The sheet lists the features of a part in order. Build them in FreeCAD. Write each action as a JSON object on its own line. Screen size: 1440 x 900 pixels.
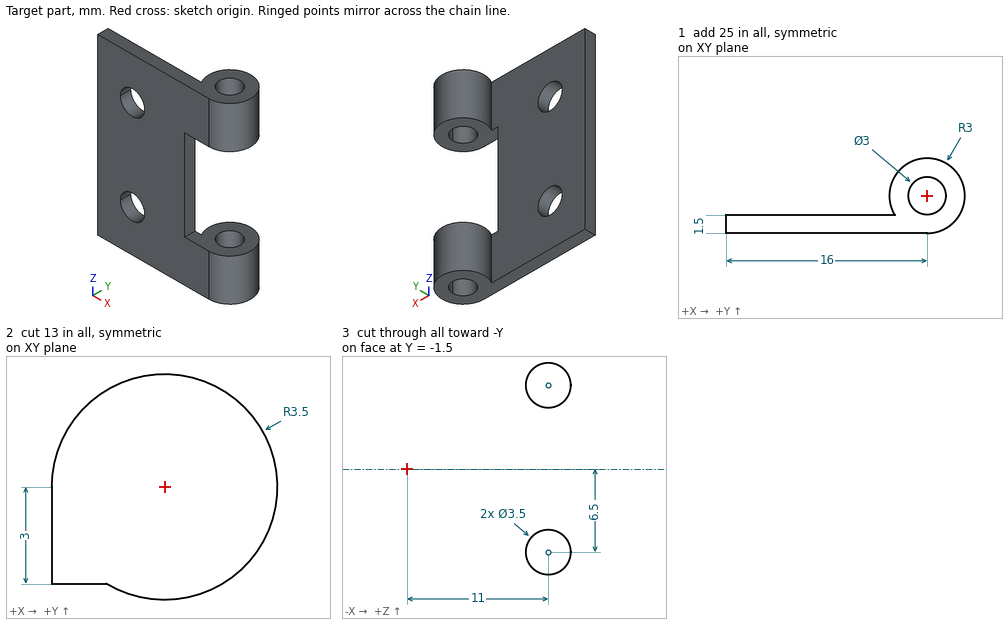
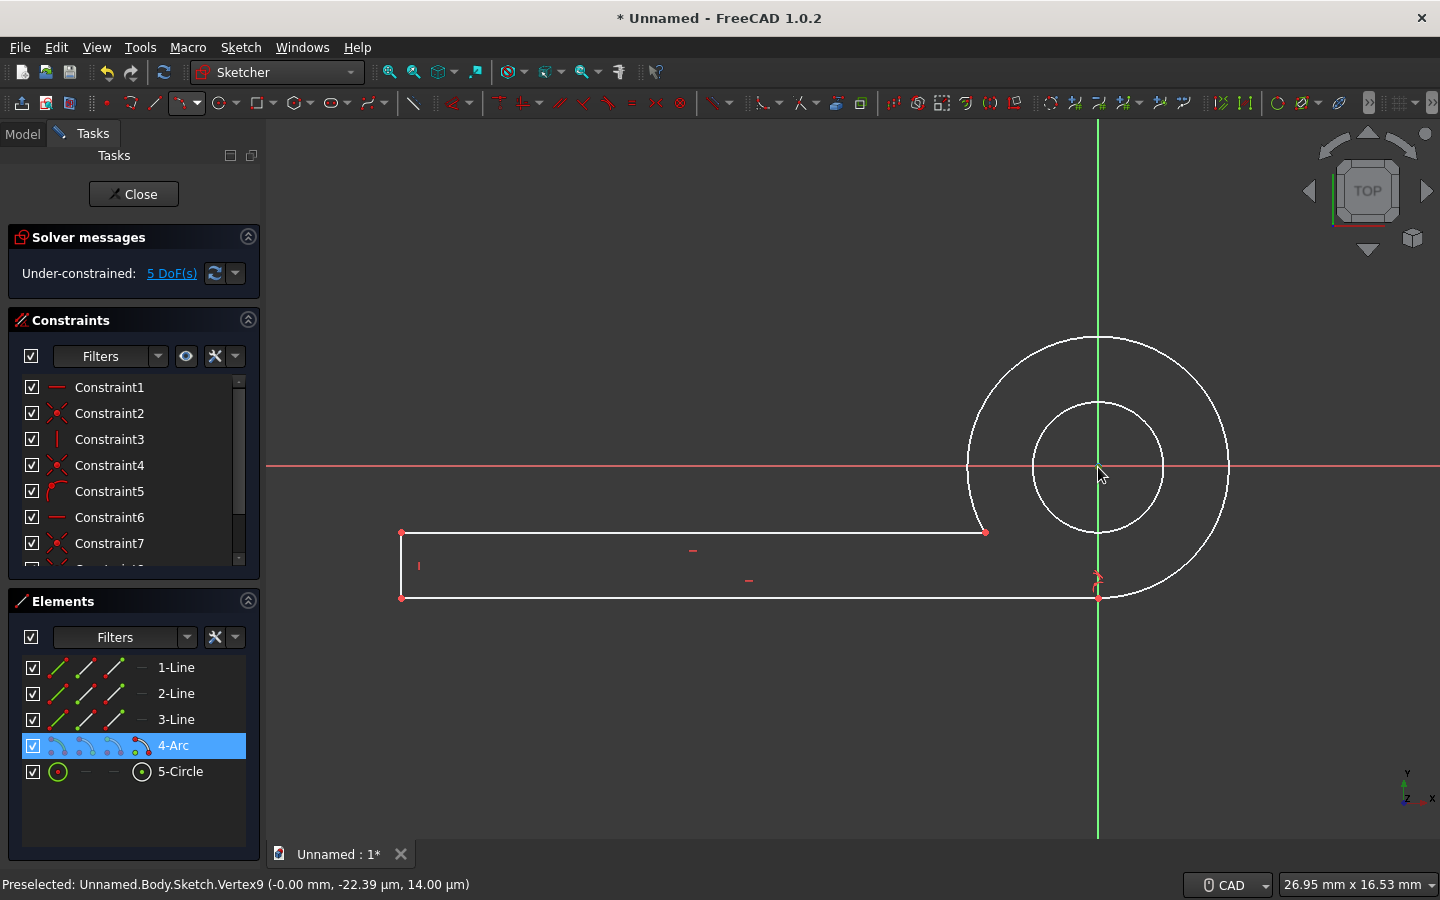
{"action": "left_click", "coordinate": [364, 466]}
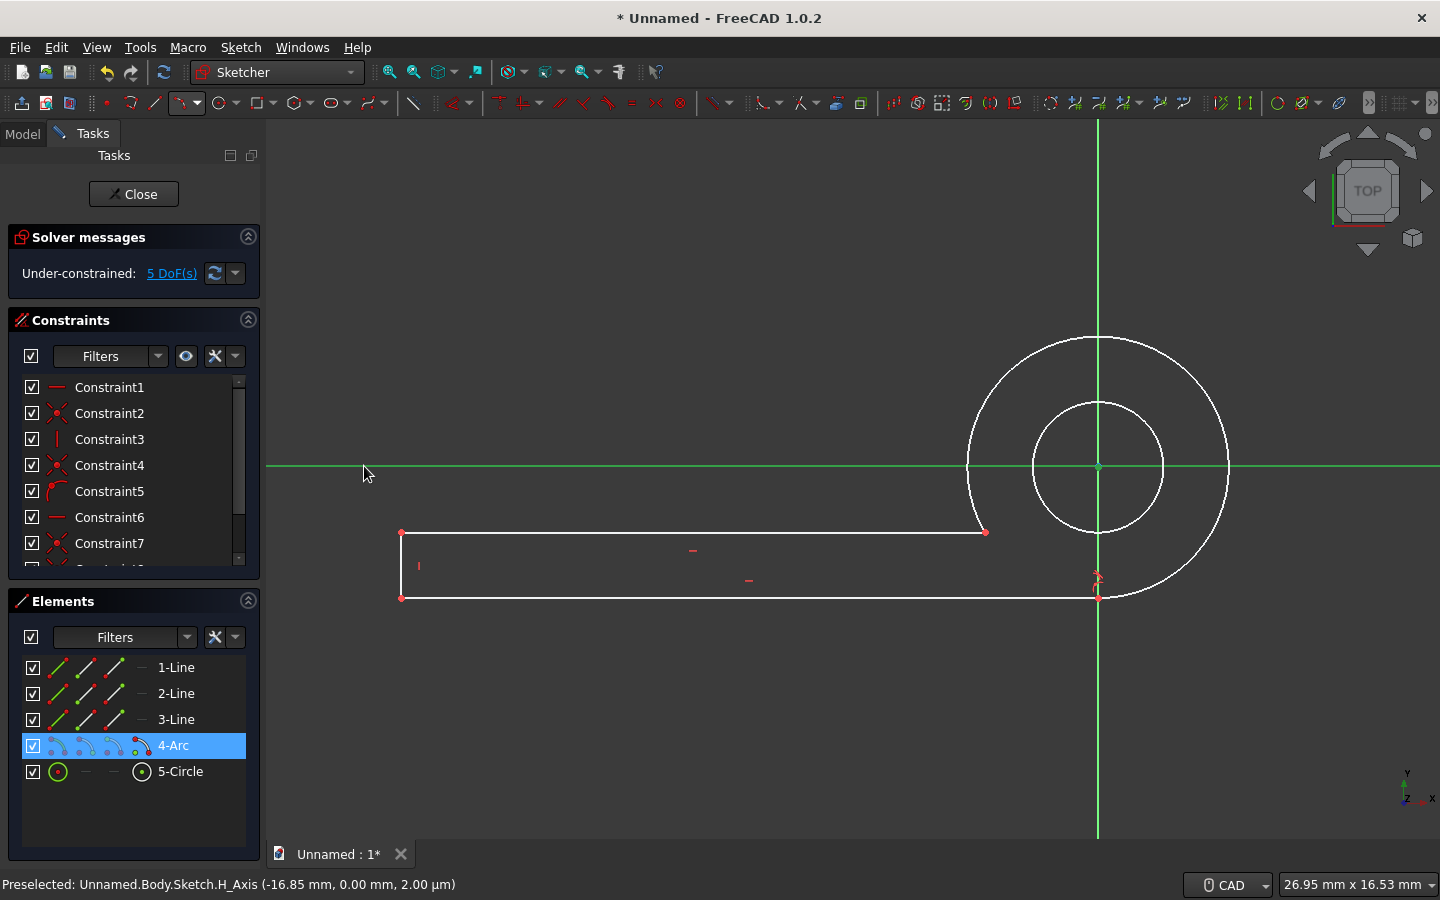
{"action": "left_click", "coordinate": [500, 104]}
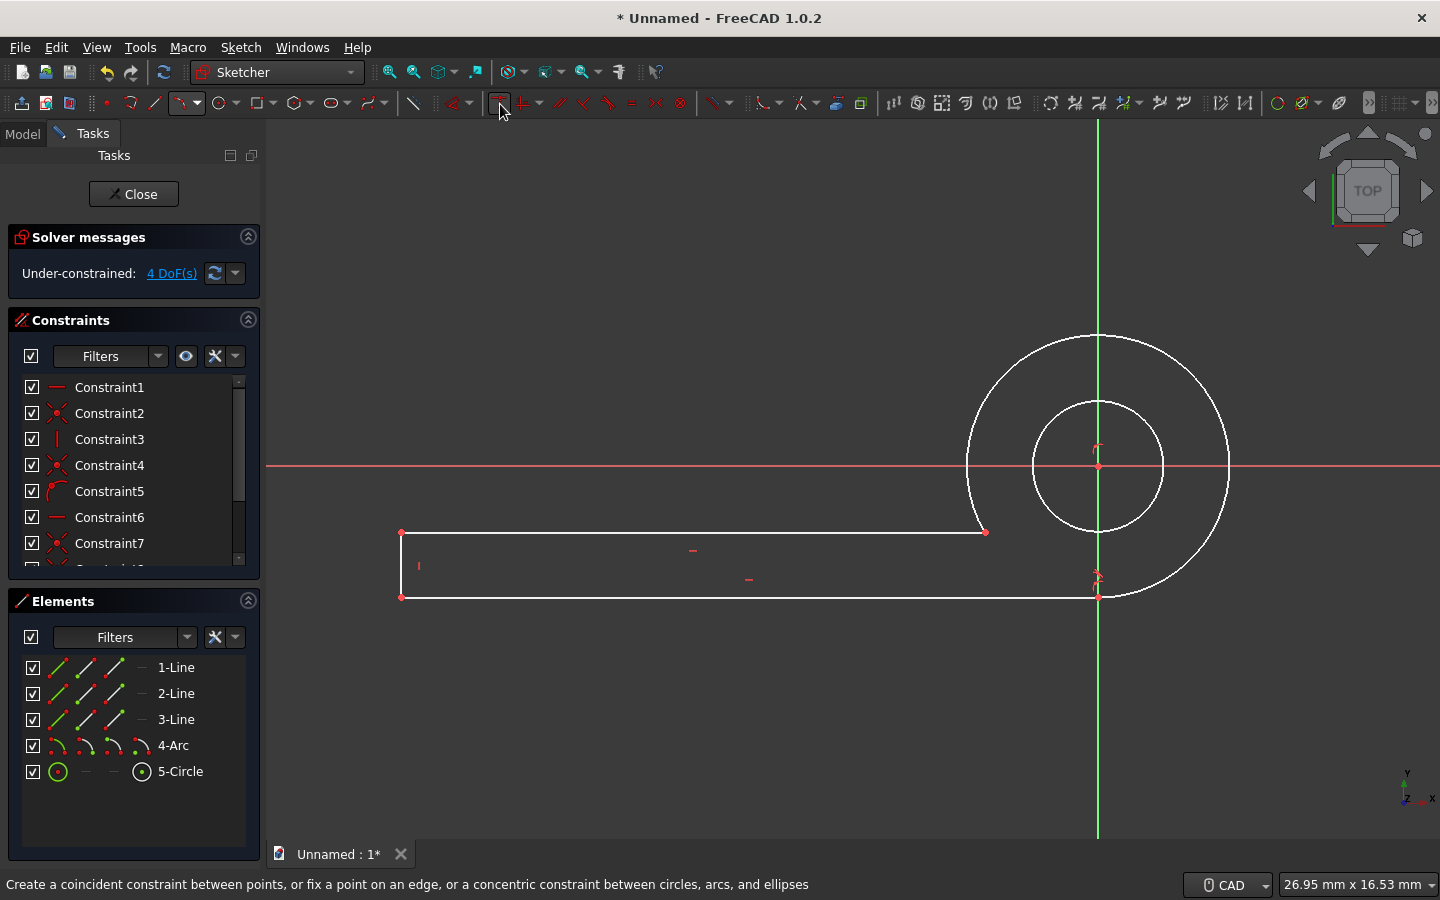
{"action": "left_click", "coordinate": [452, 104]}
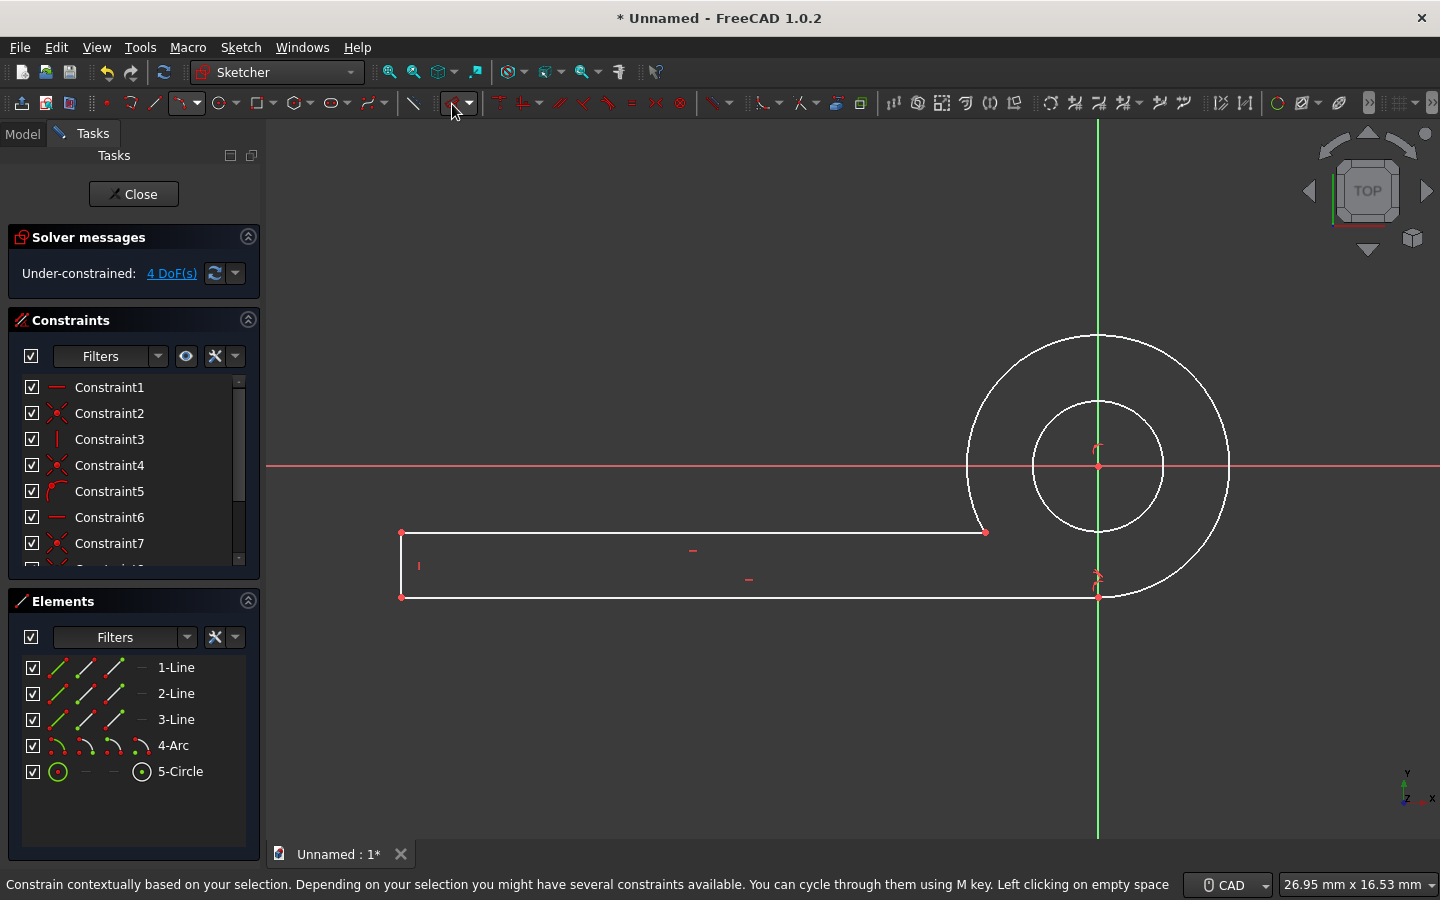
{"action": "left_click", "coordinate": [1229, 466]}
{"action": "left_click", "coordinate": [1241, 544]}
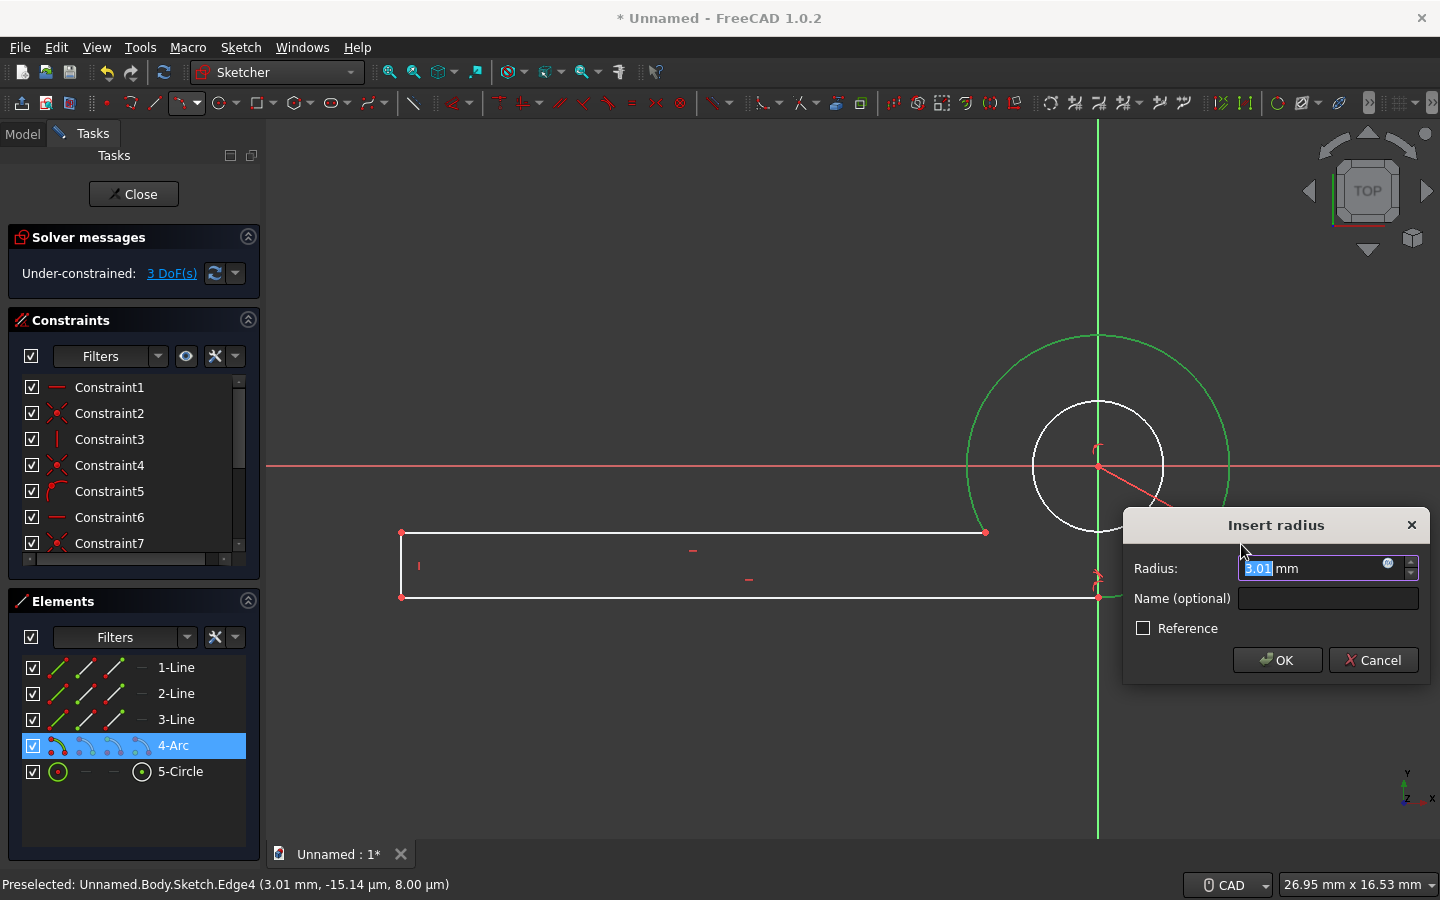
{"action": "type", "text": "3"}
{"action": "key", "text": "Return"}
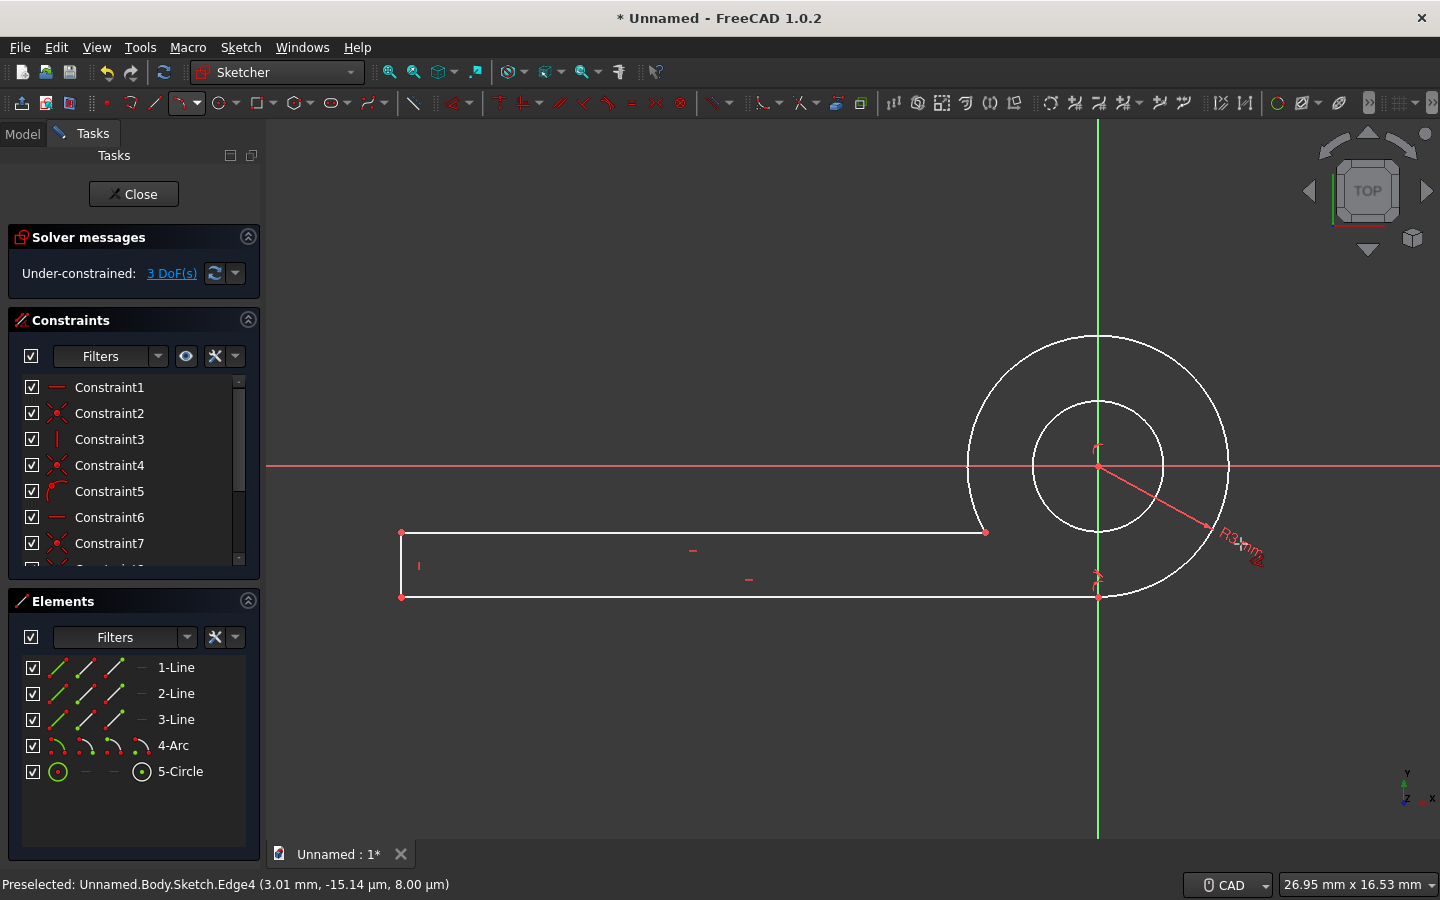
{"action": "left_click", "coordinate": [1144, 420]}
{"action": "left_click", "coordinate": [1167, 397]}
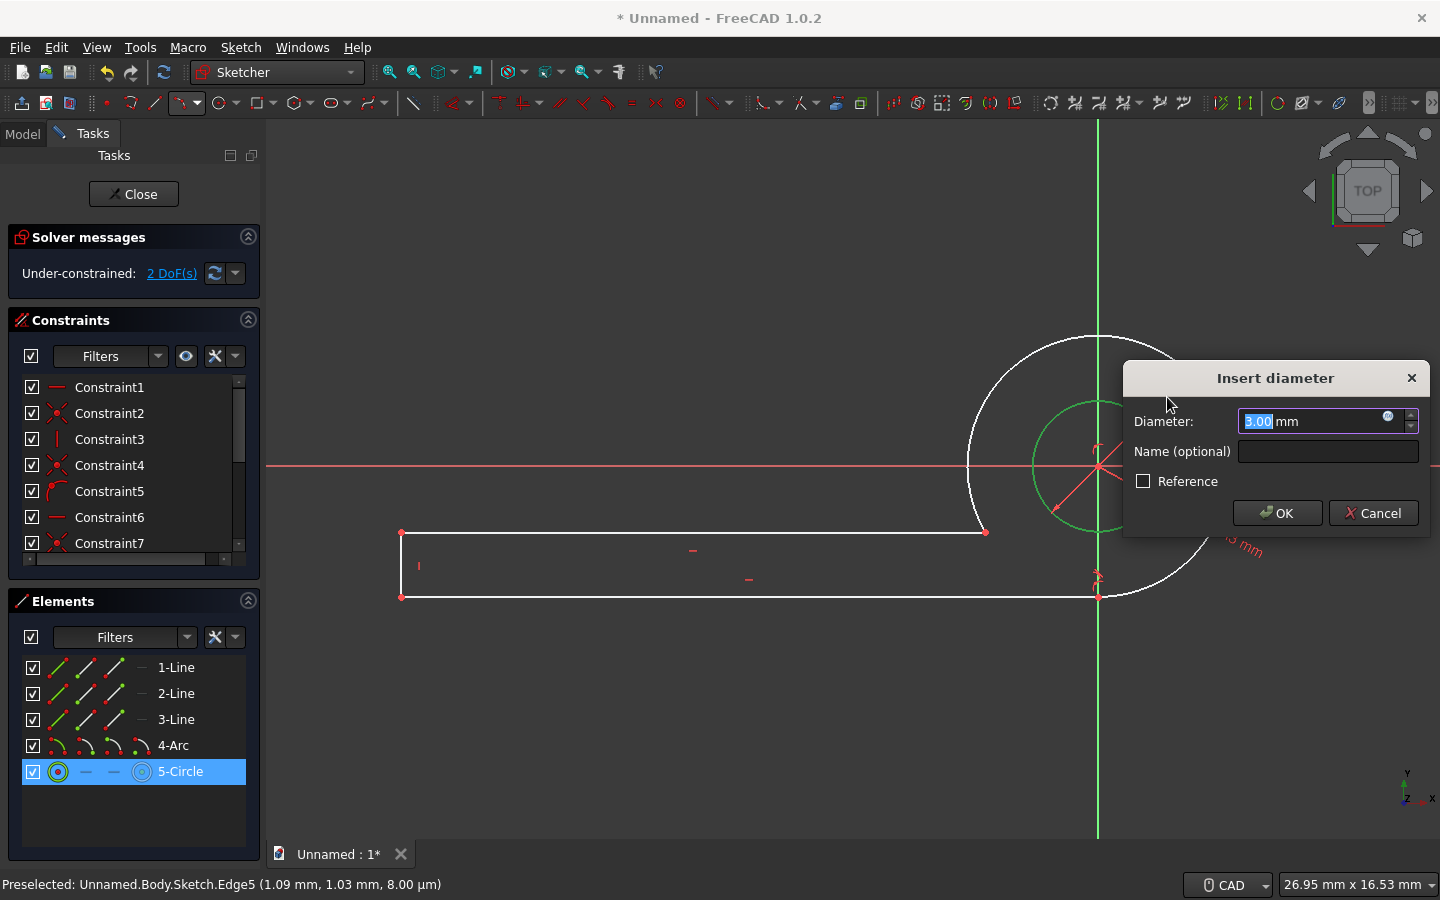
{"action": "type", "text": "3"}
{"action": "key", "text": "Return"}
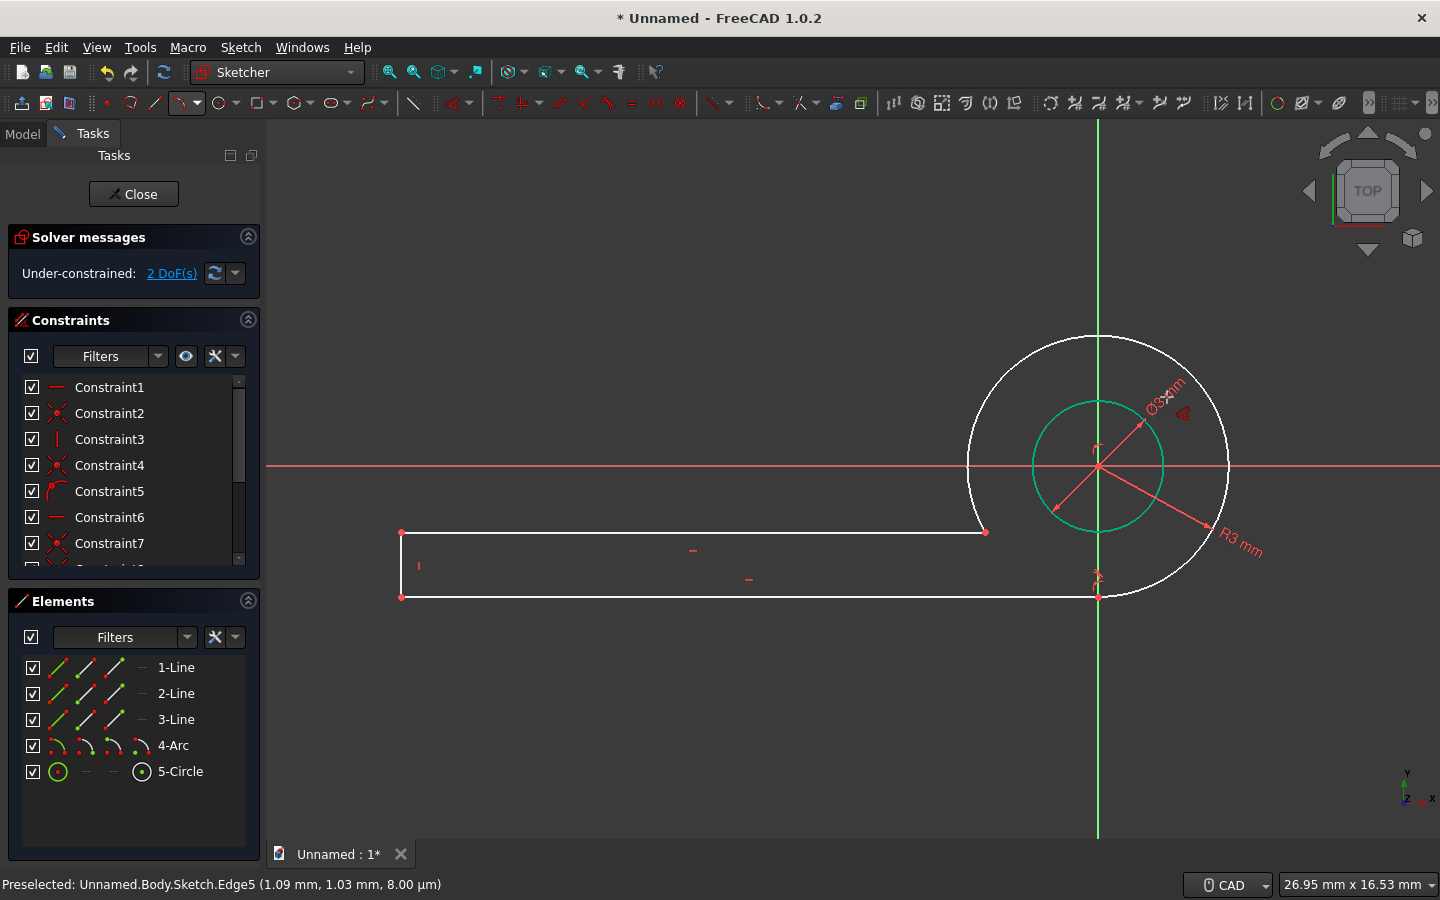
{"action": "left_click", "coordinate": [610, 597]}
{"action": "left_click", "coordinate": [750, 631]}